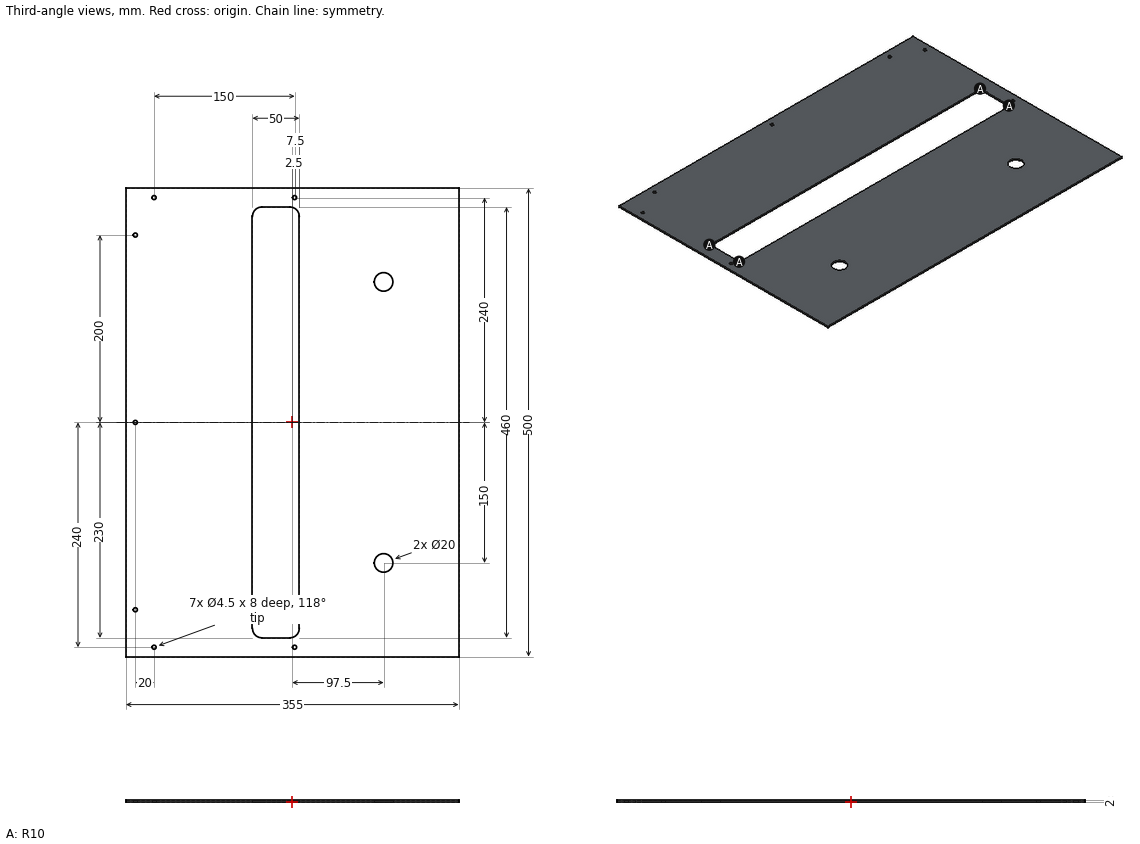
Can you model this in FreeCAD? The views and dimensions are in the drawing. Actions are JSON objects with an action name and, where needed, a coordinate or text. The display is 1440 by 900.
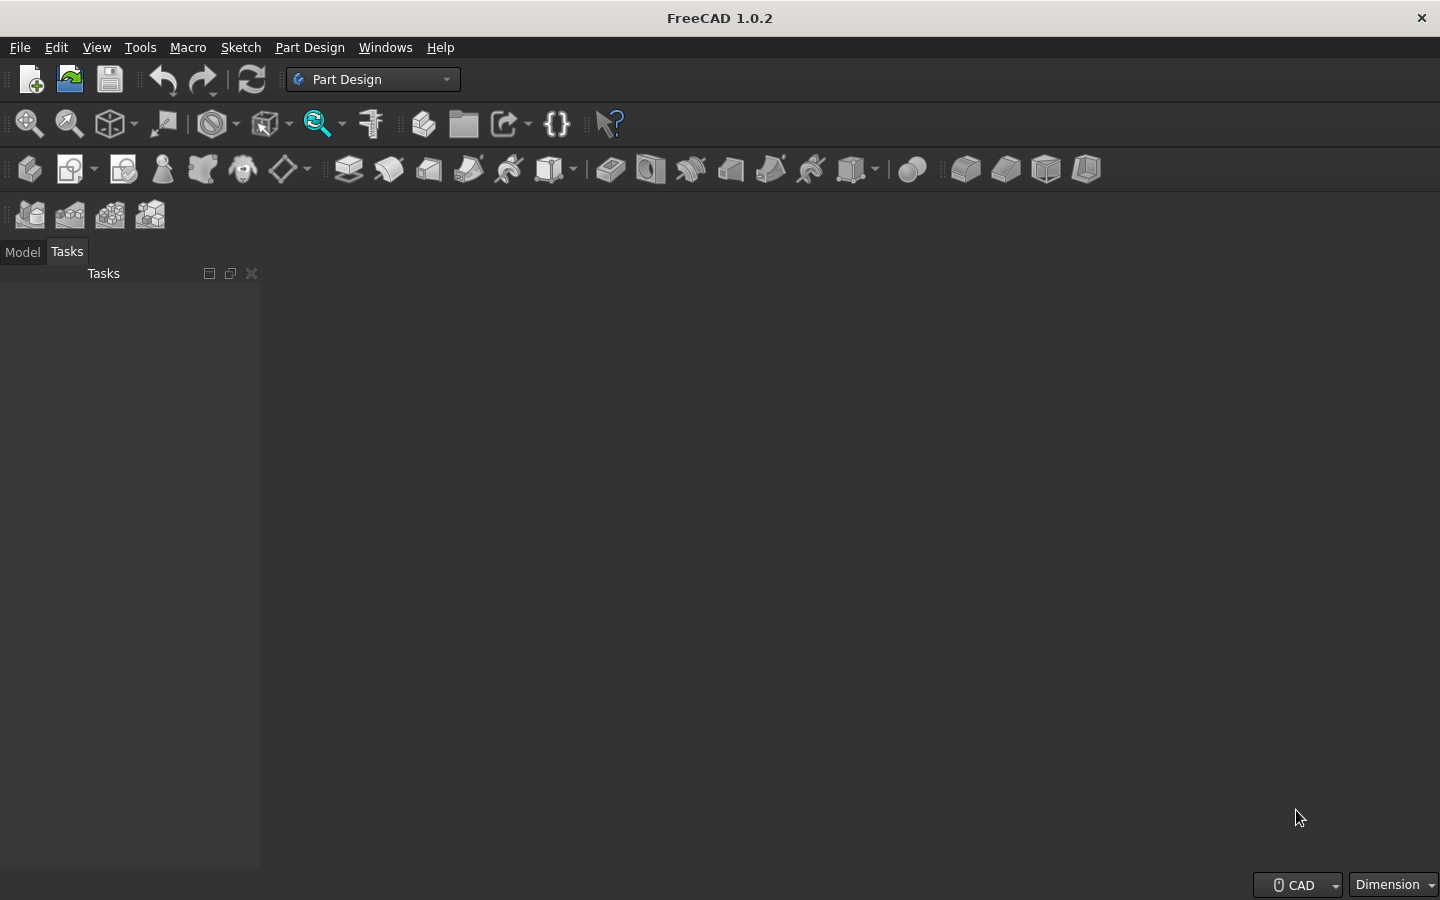
{"action": "left_click", "coordinate": [30, 80]}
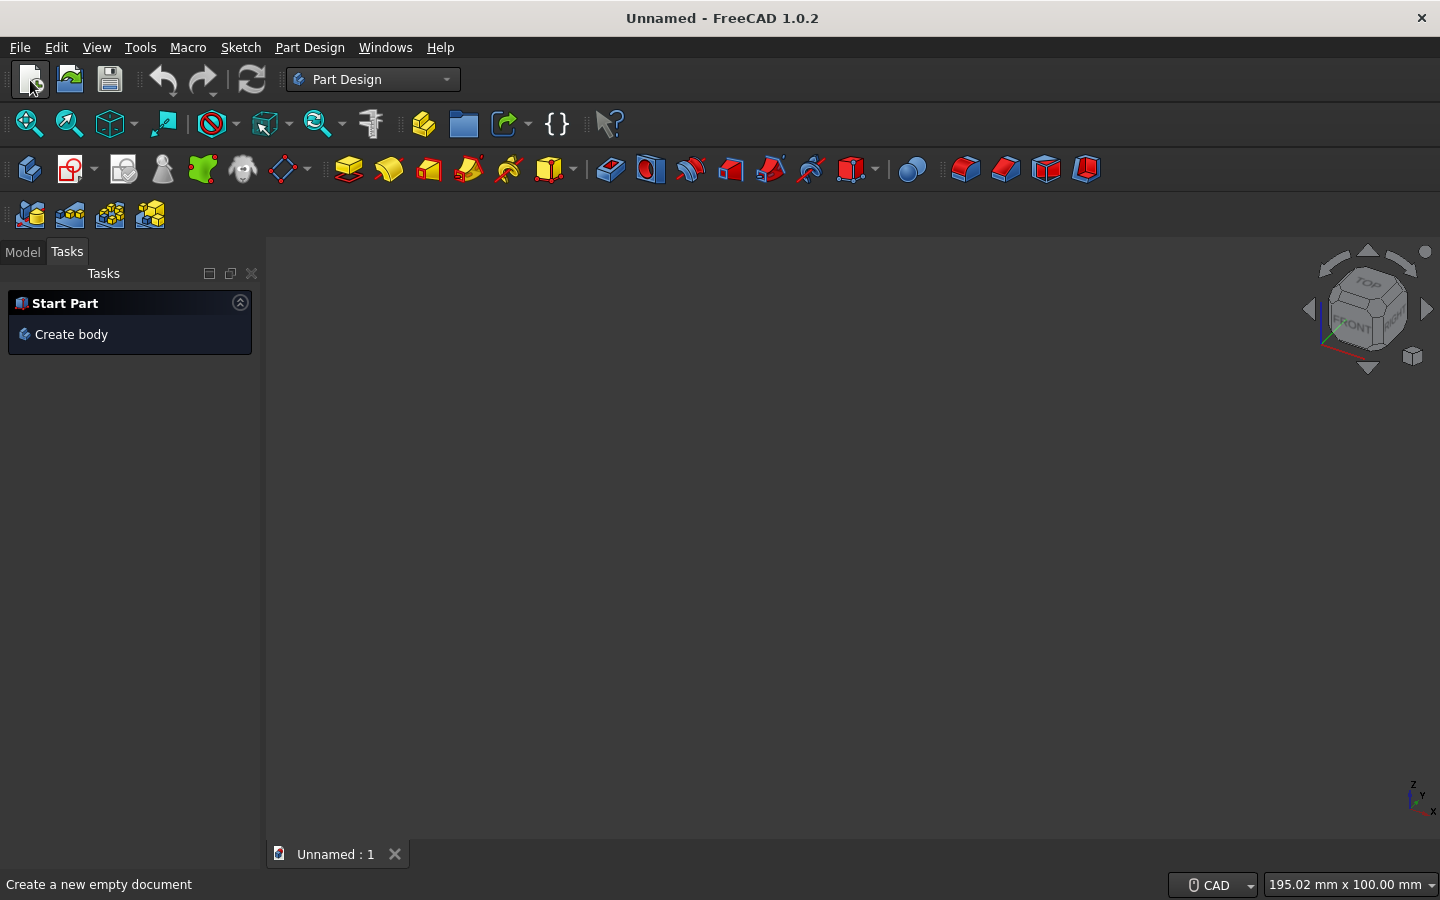
{"action": "left_click", "coordinate": [70, 170]}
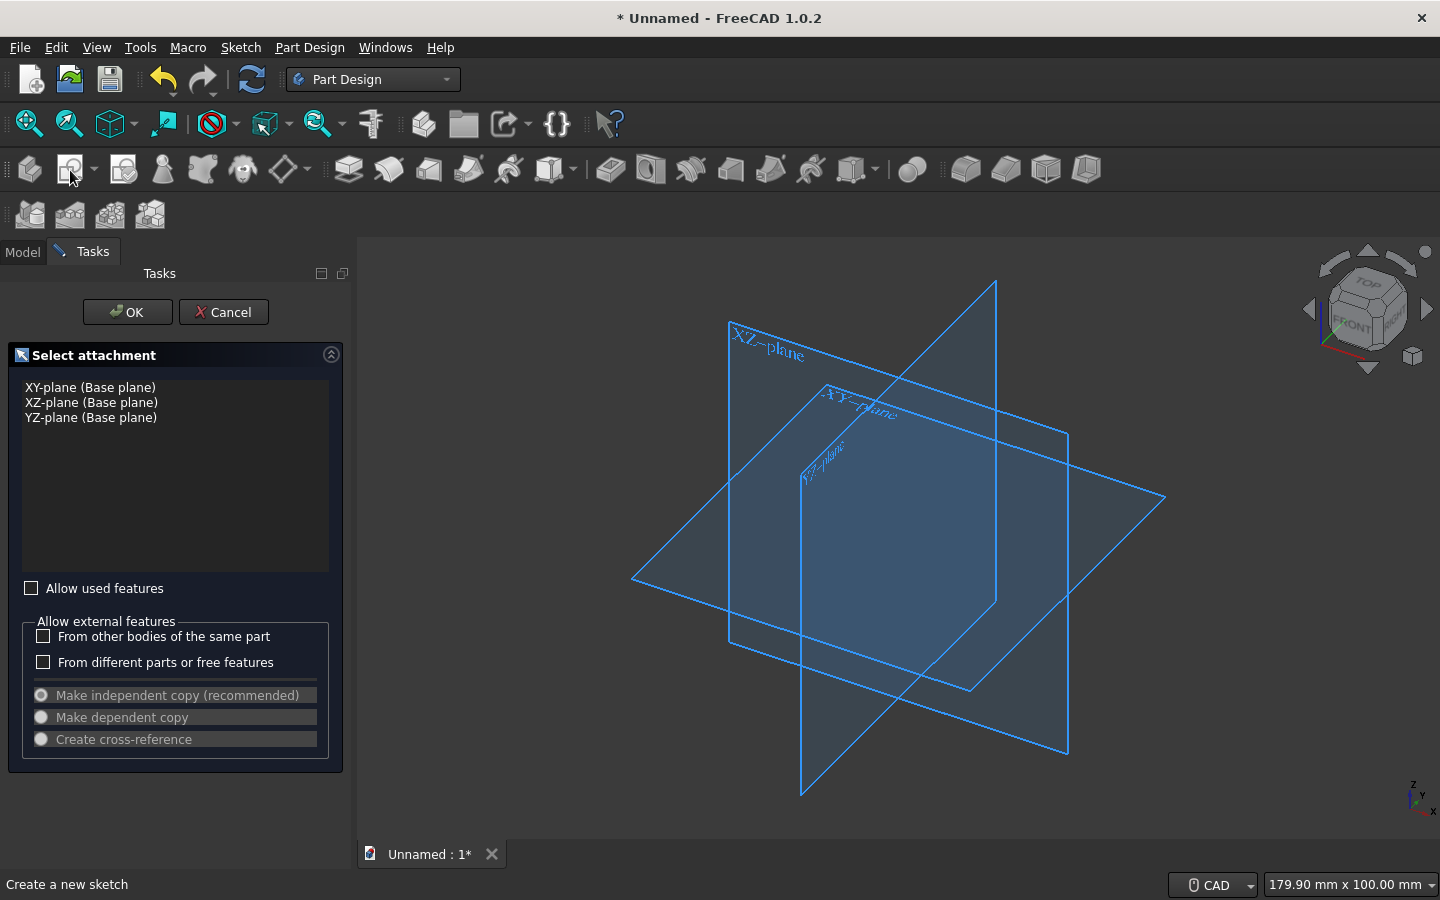
{"action": "left_click", "coordinate": [82, 388]}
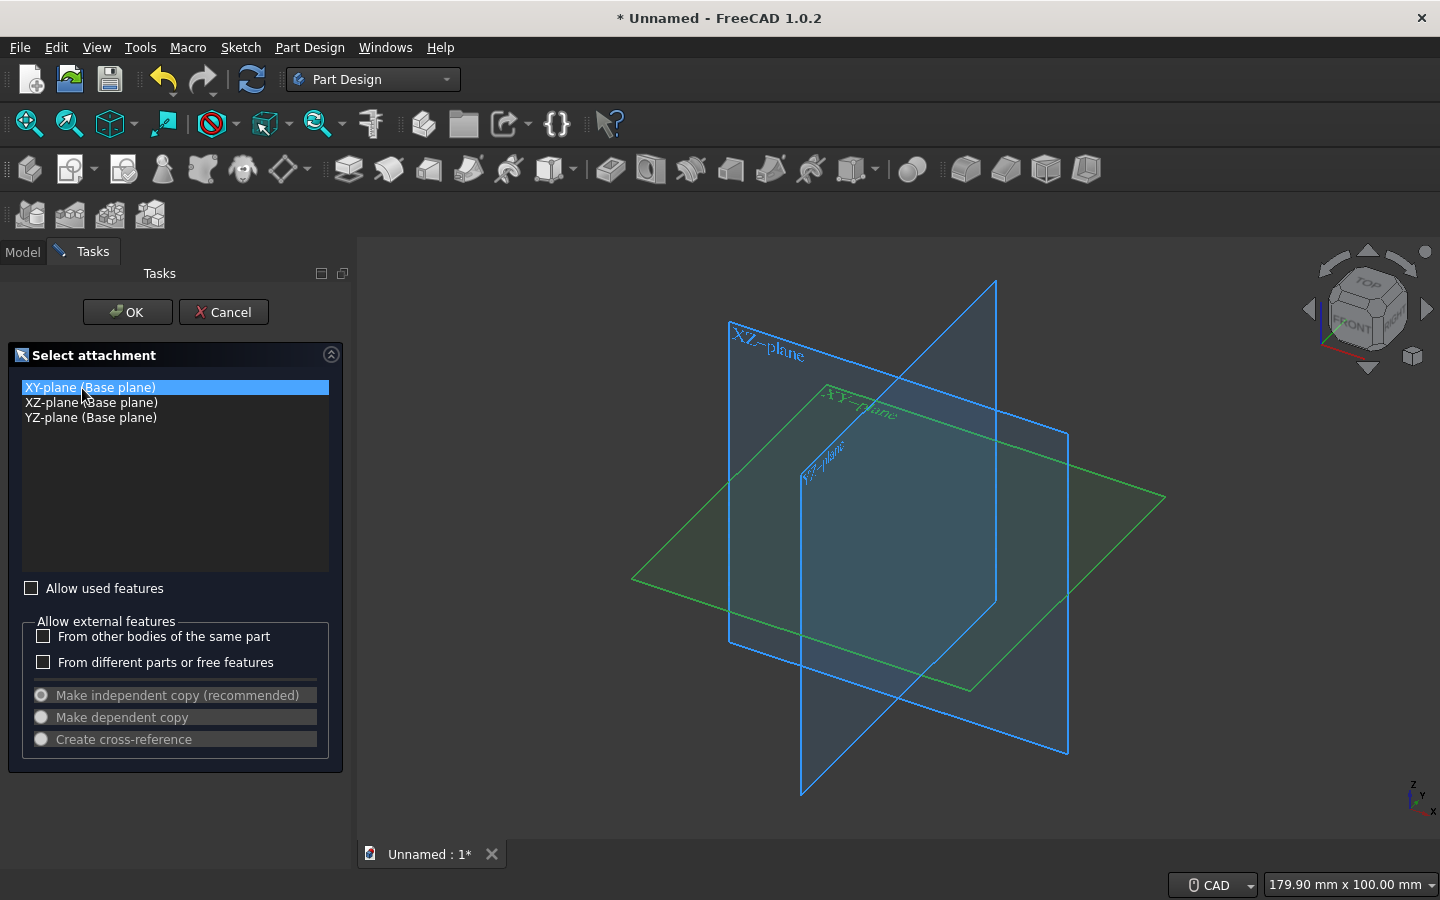
{"action": "left_click", "coordinate": [128, 312]}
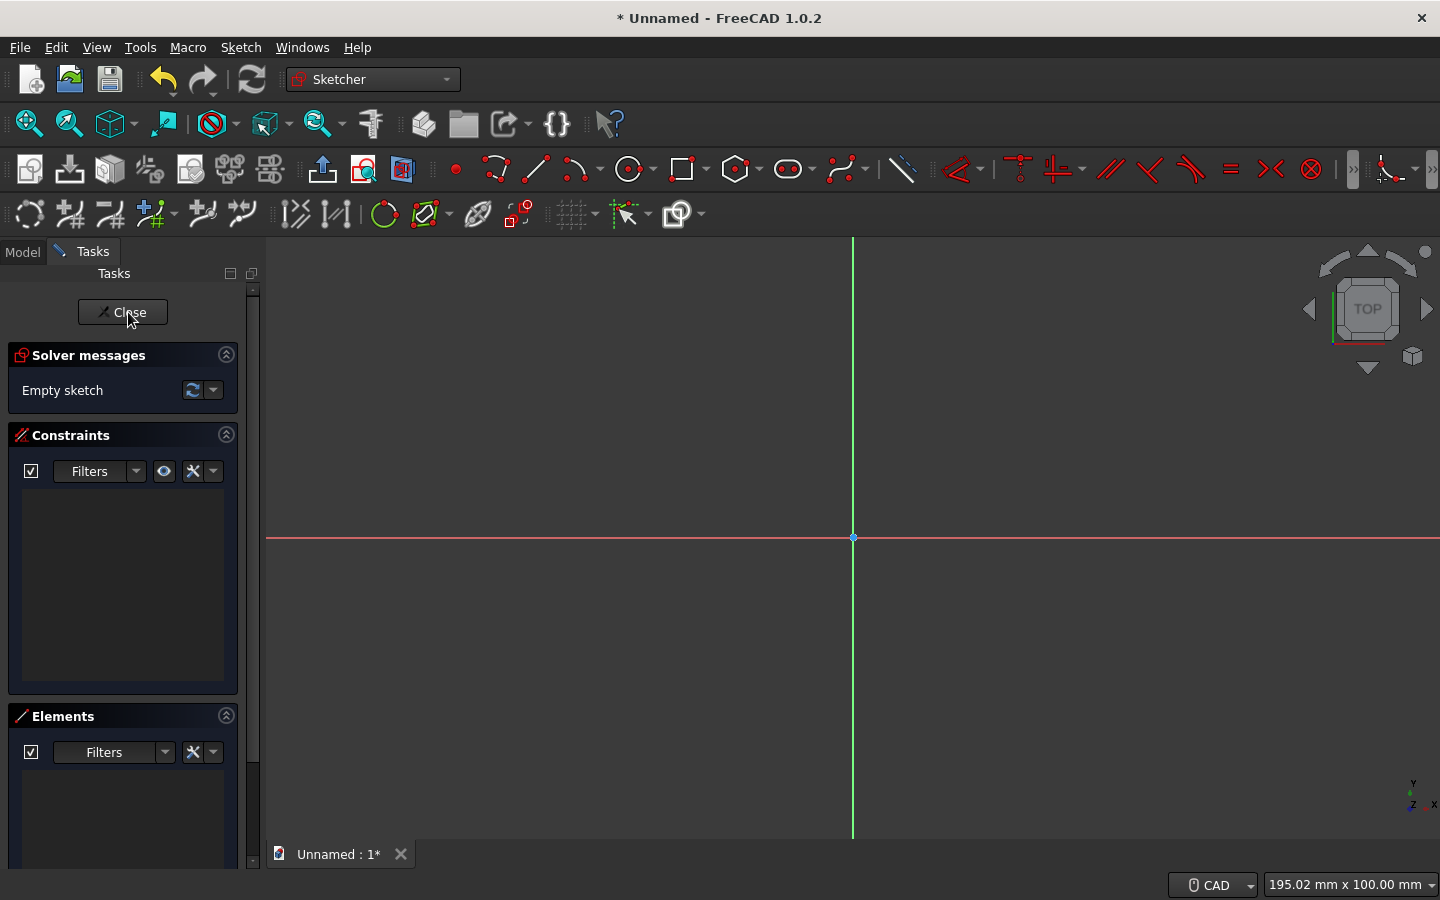
{"action": "scroll", "coordinate": [774, 538], "scroll_direction": "down", "scroll_amount": 10}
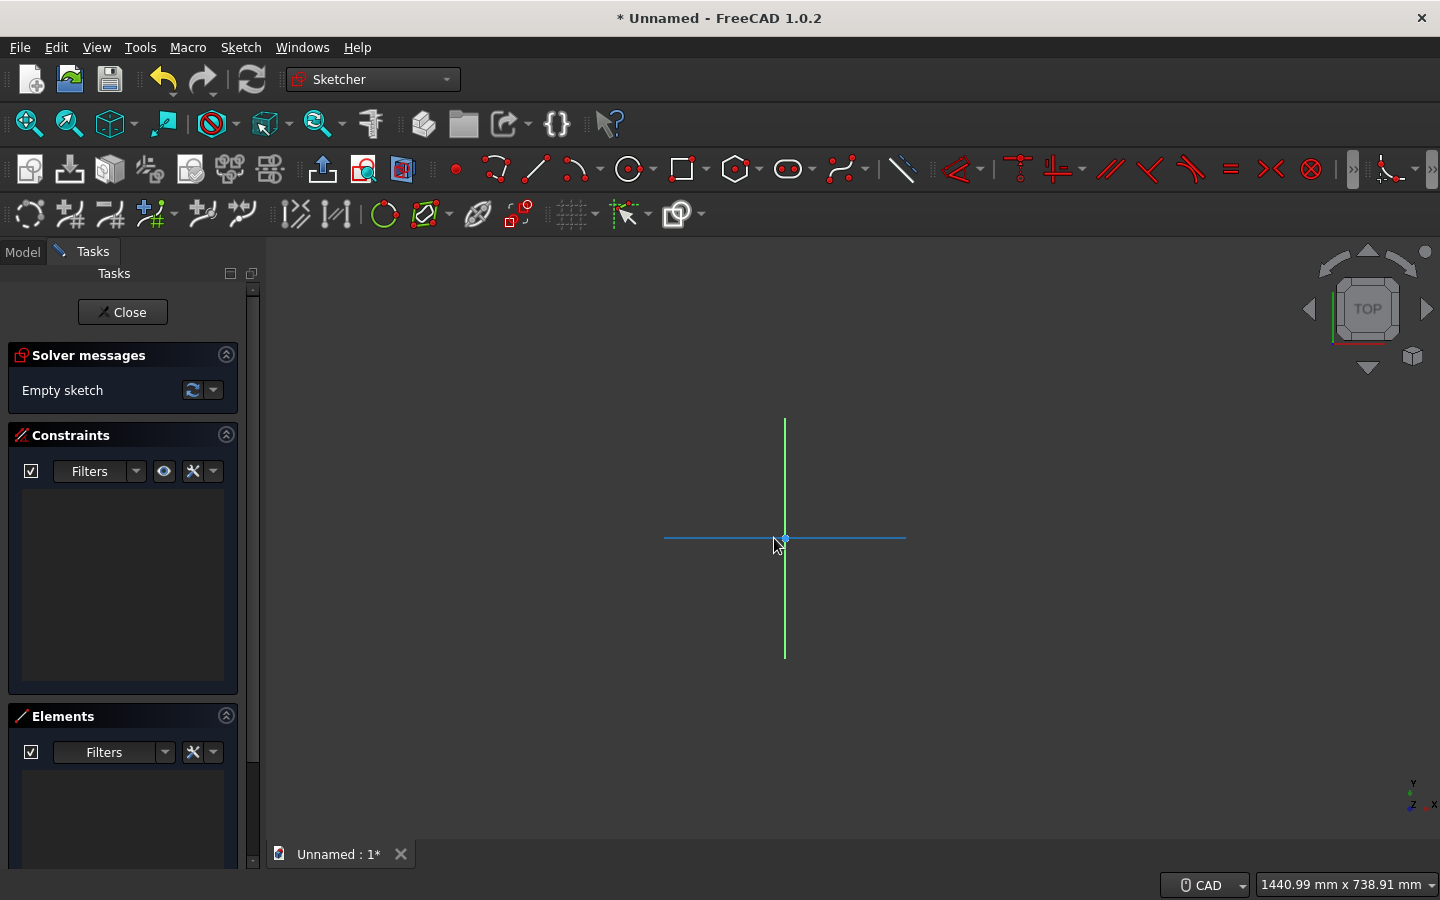
{"action": "key", "text": "g v"}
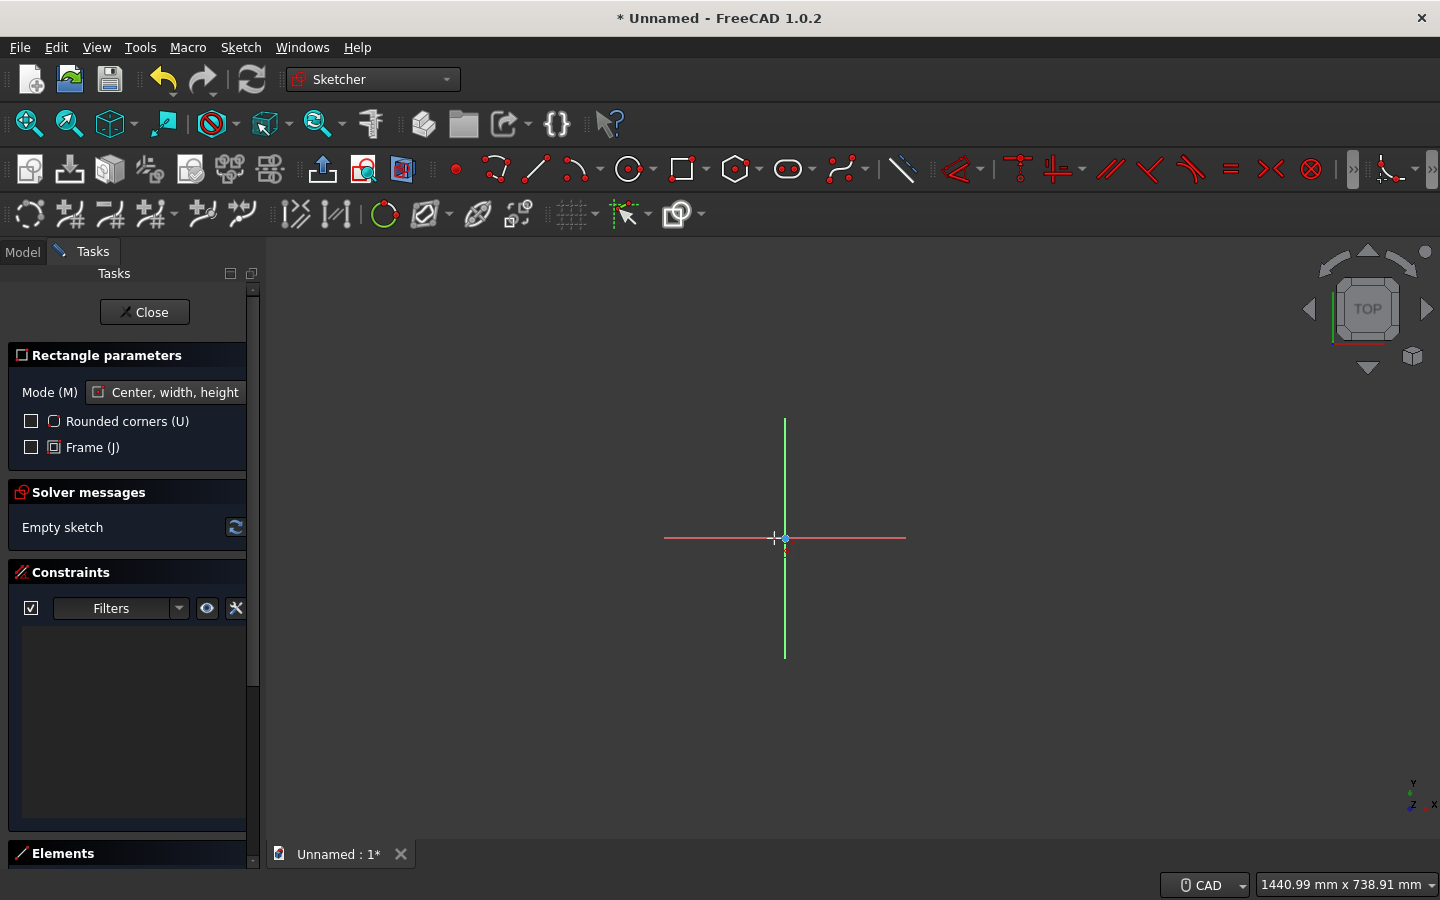
{"action": "left_click", "coordinate": [785, 538]}
{"action": "mouse_move", "coordinate": [930, 335]}